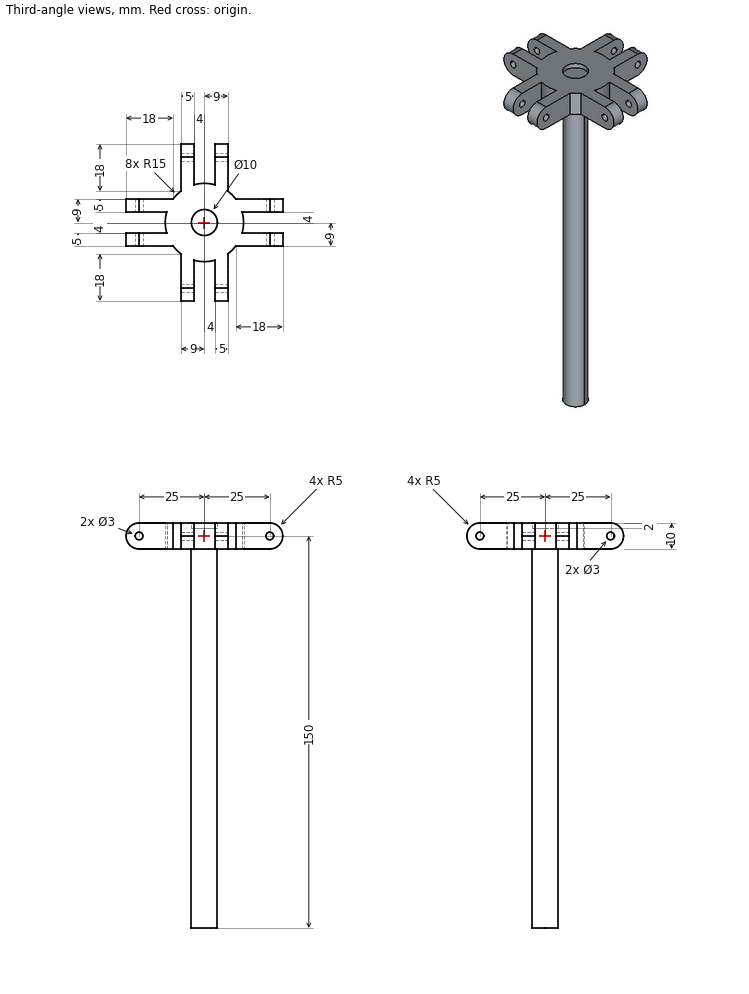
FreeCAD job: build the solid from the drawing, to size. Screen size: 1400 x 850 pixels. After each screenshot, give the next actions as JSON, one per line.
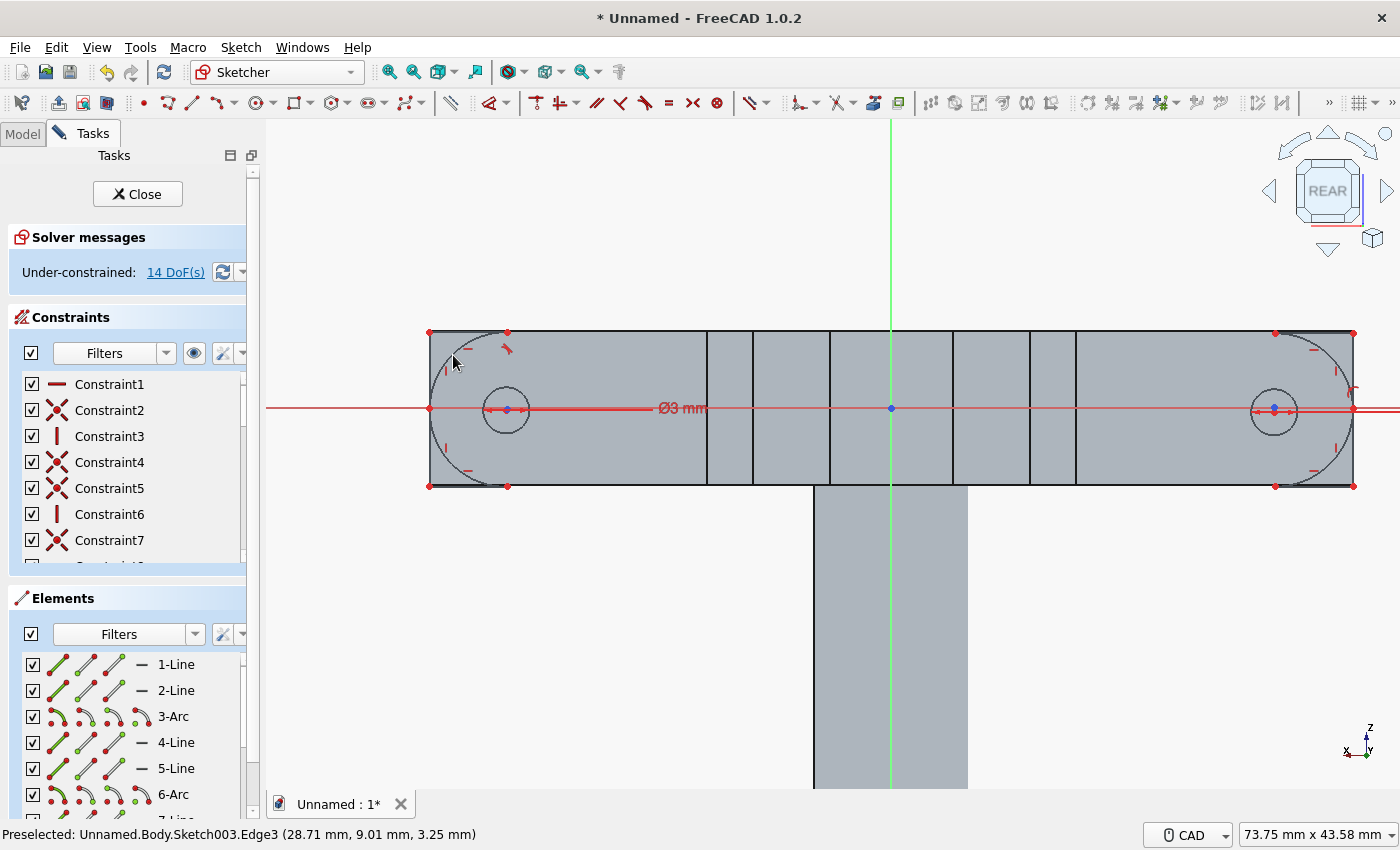
{"action": "left_click", "coordinate": [430, 355]}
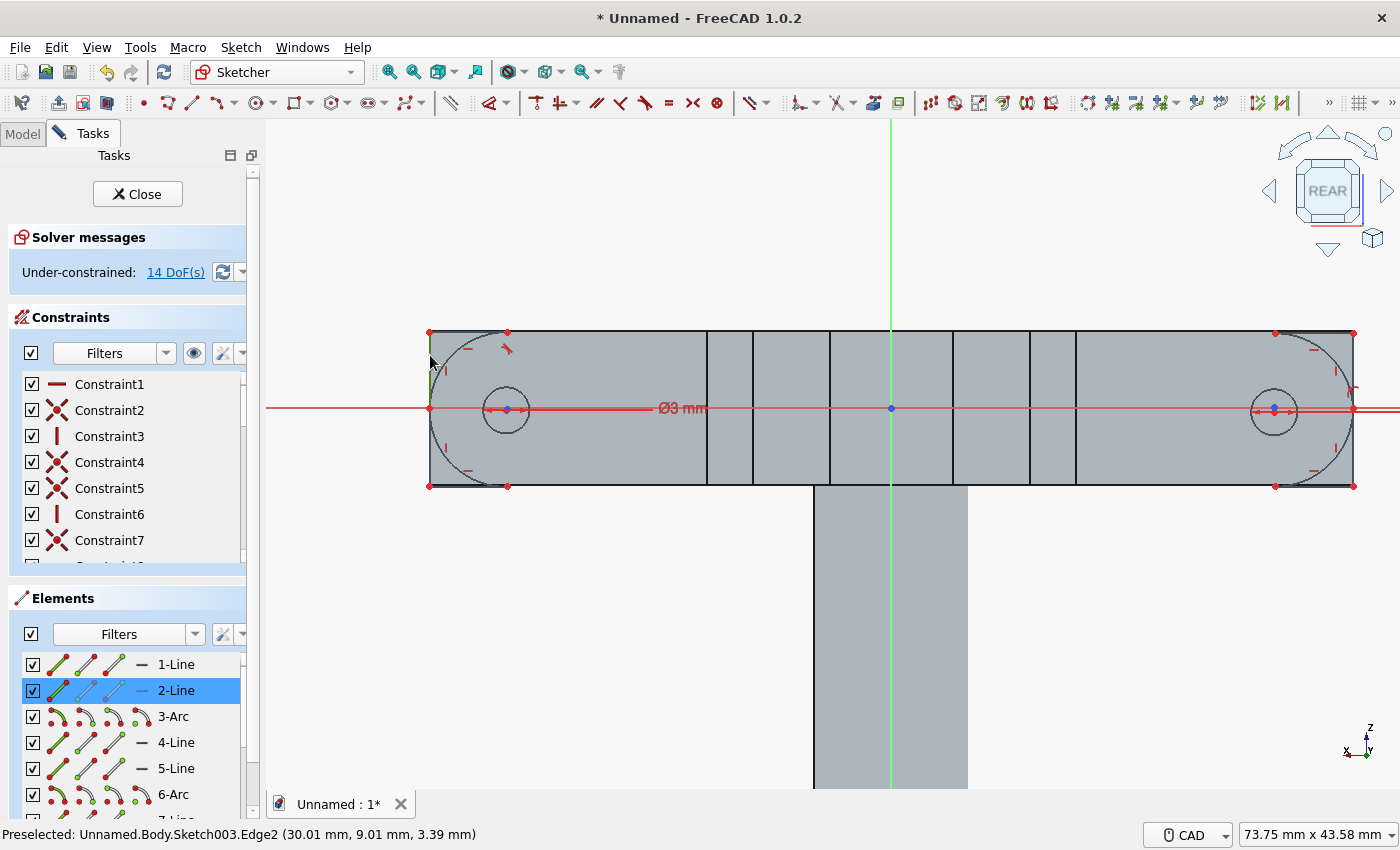
{"action": "left_click", "coordinate": [453, 354]}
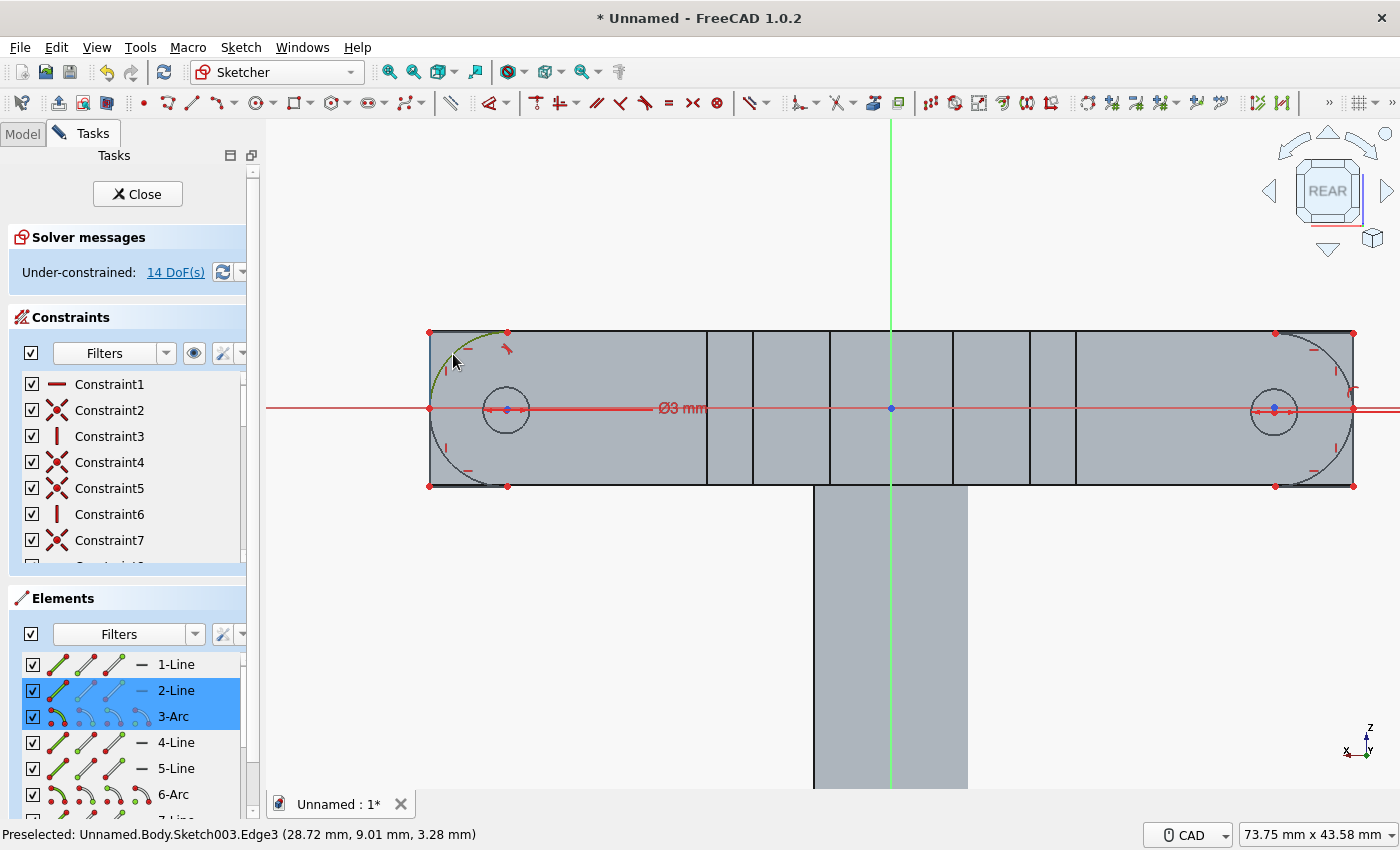
{"action": "key", "text": "t"}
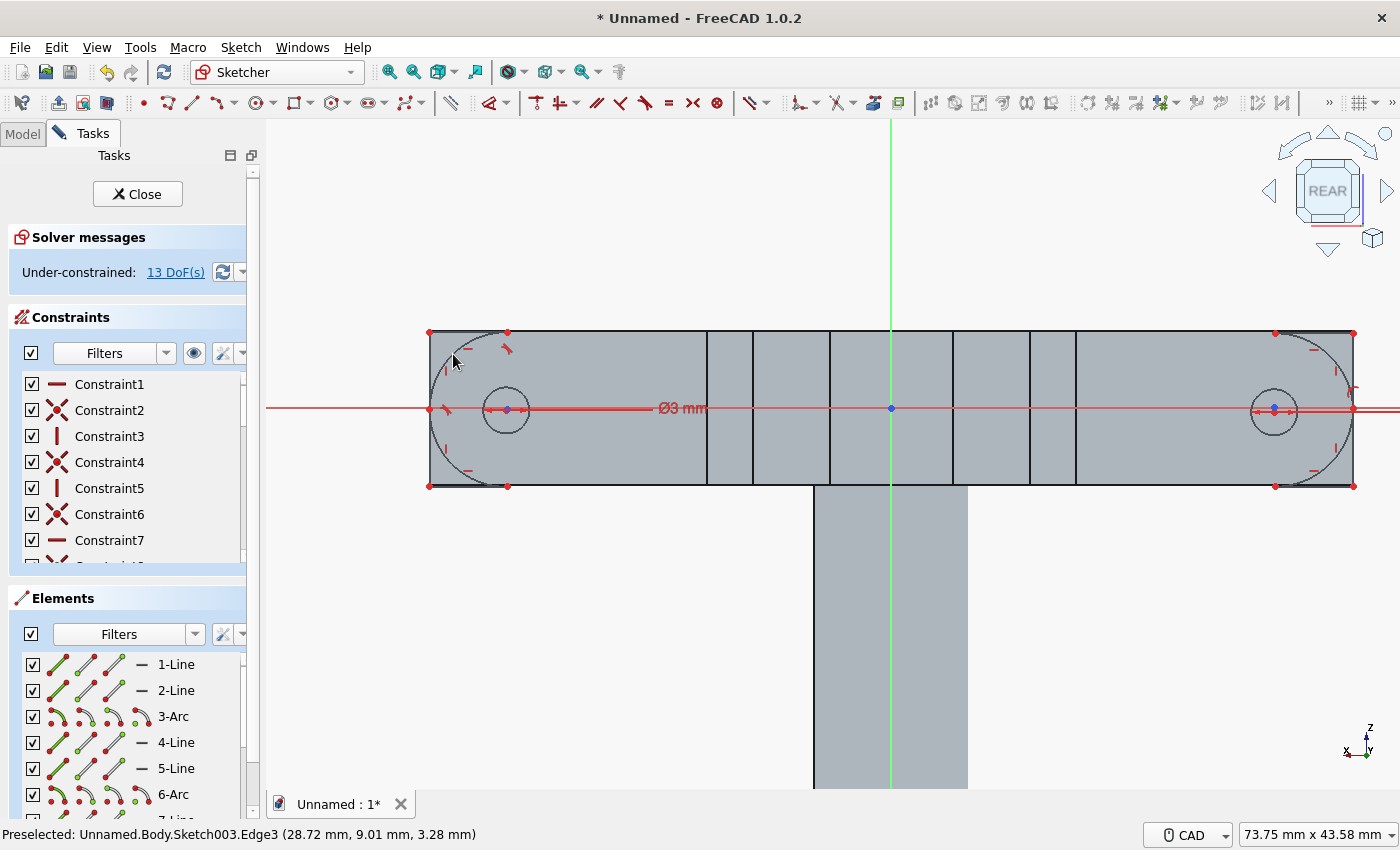
{"action": "left_click", "coordinate": [430, 355]}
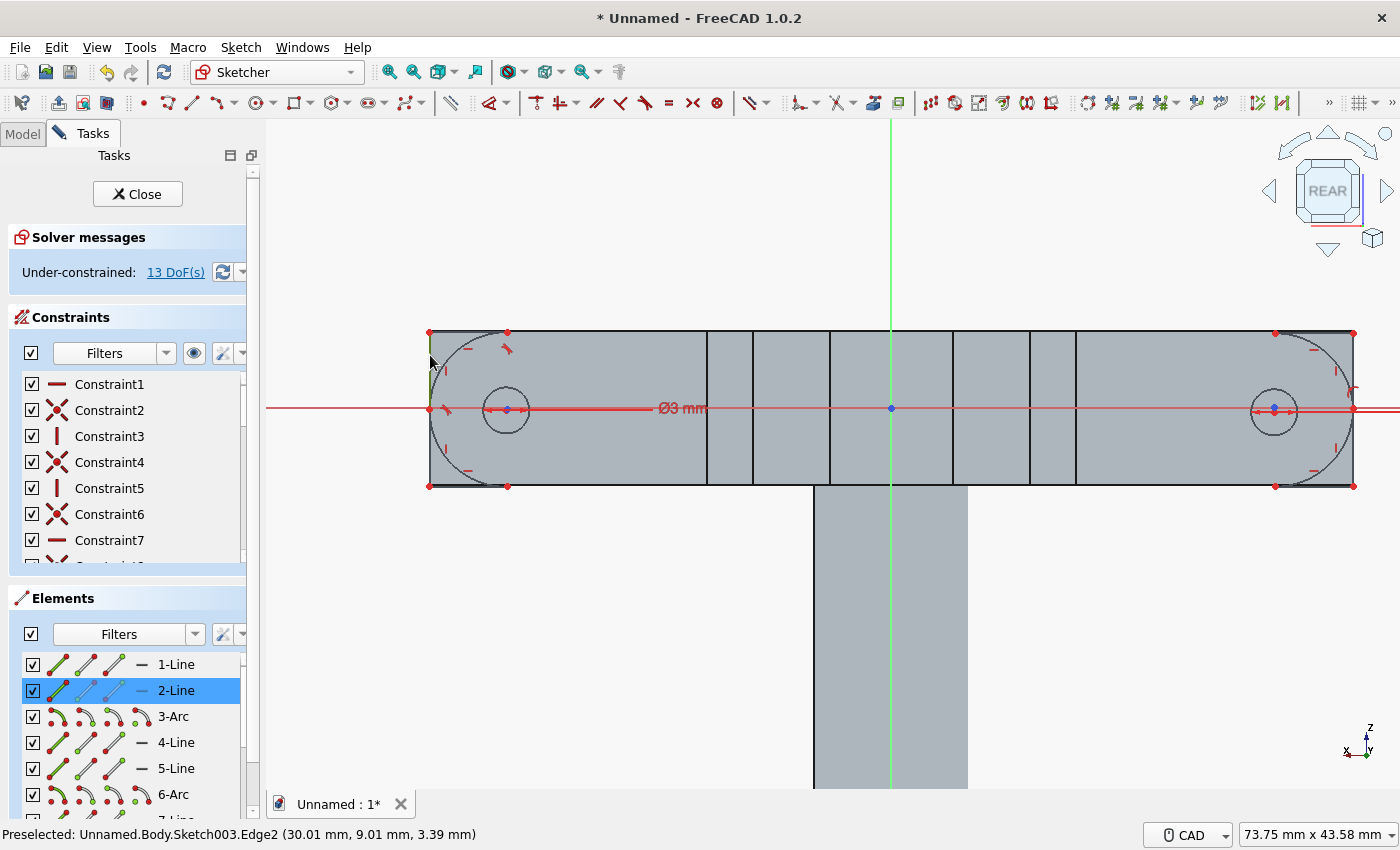
{"action": "left_click", "coordinate": [452, 465]}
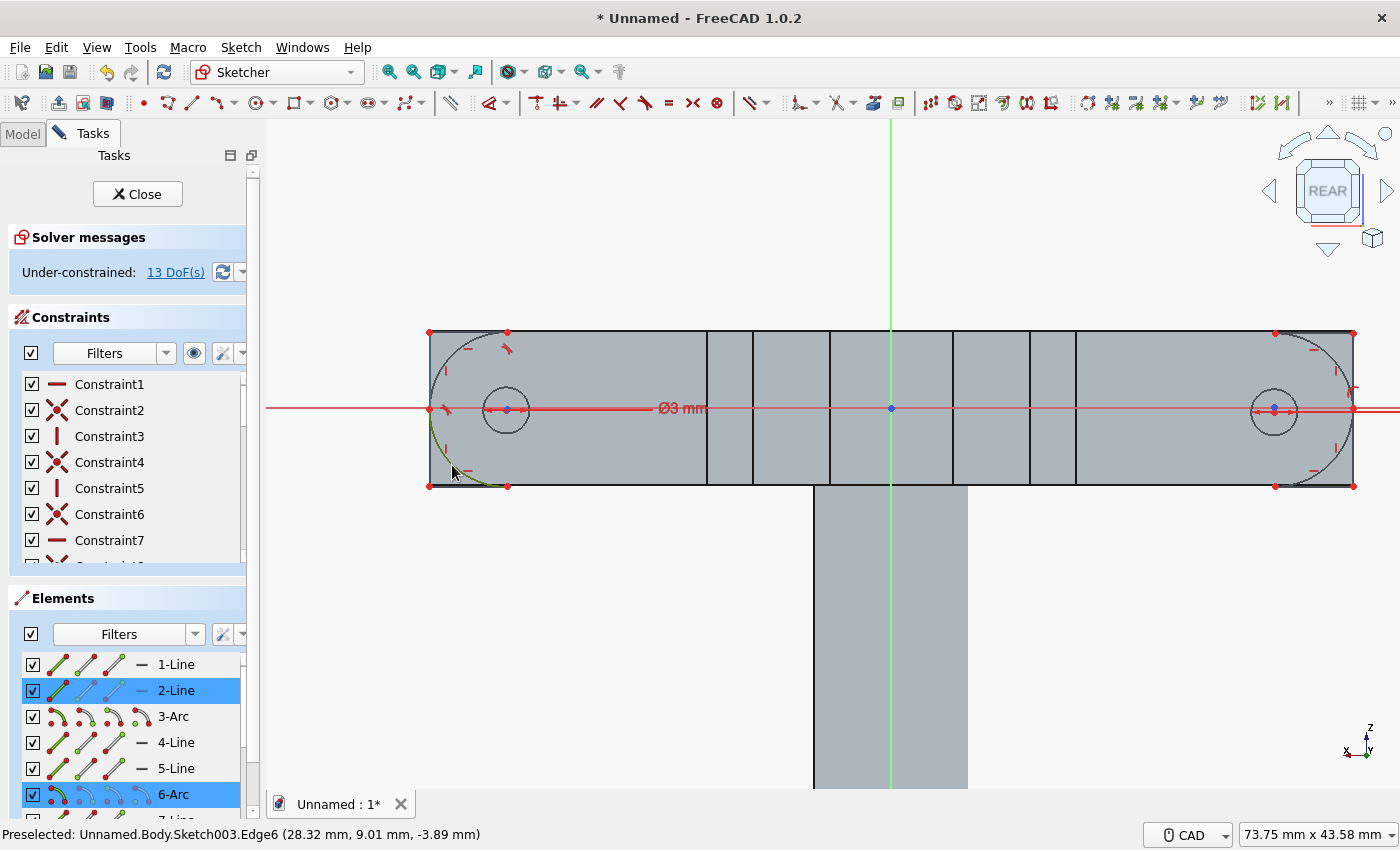
{"action": "key", "text": "t"}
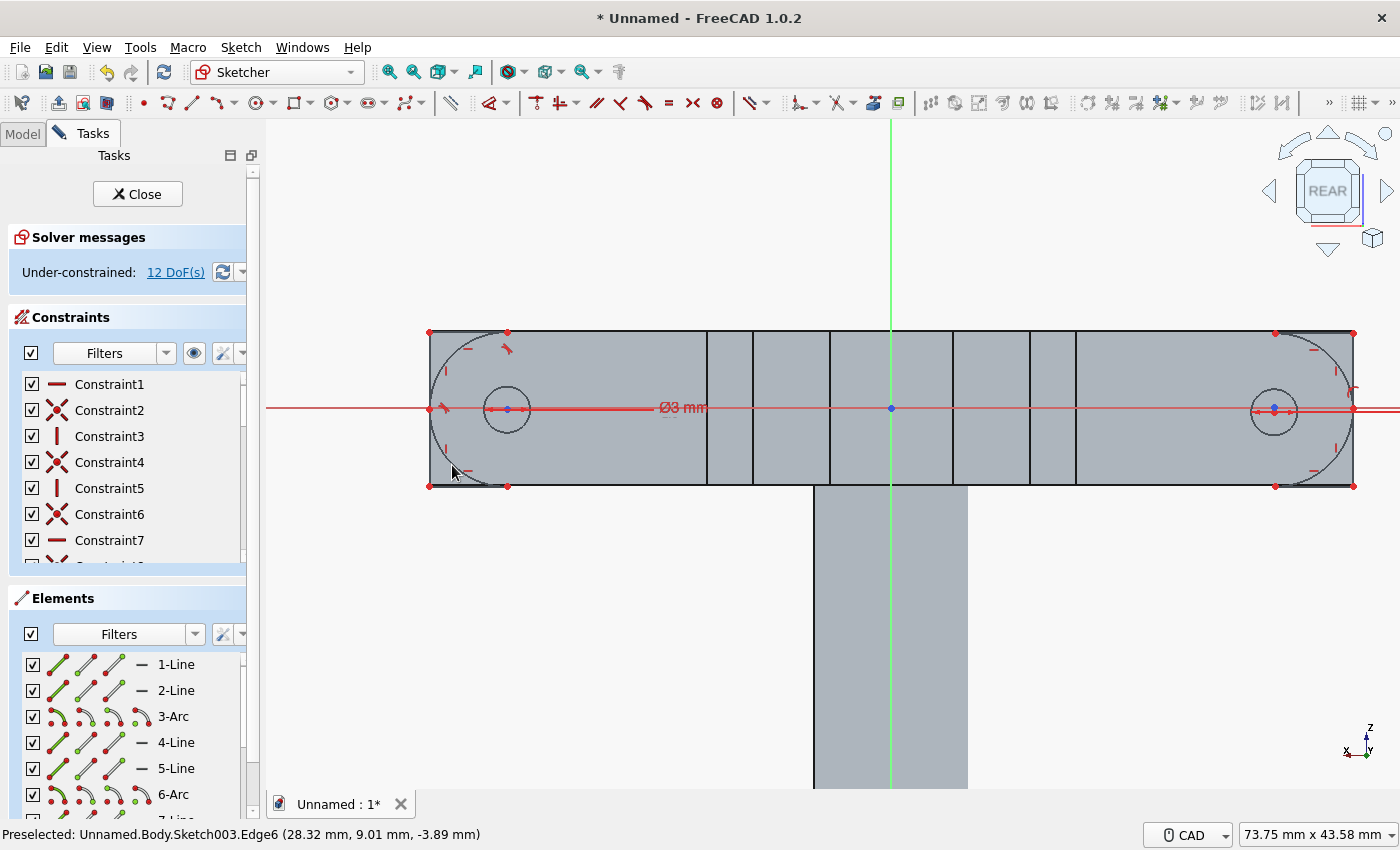
{"action": "left_click", "coordinate": [453, 487]}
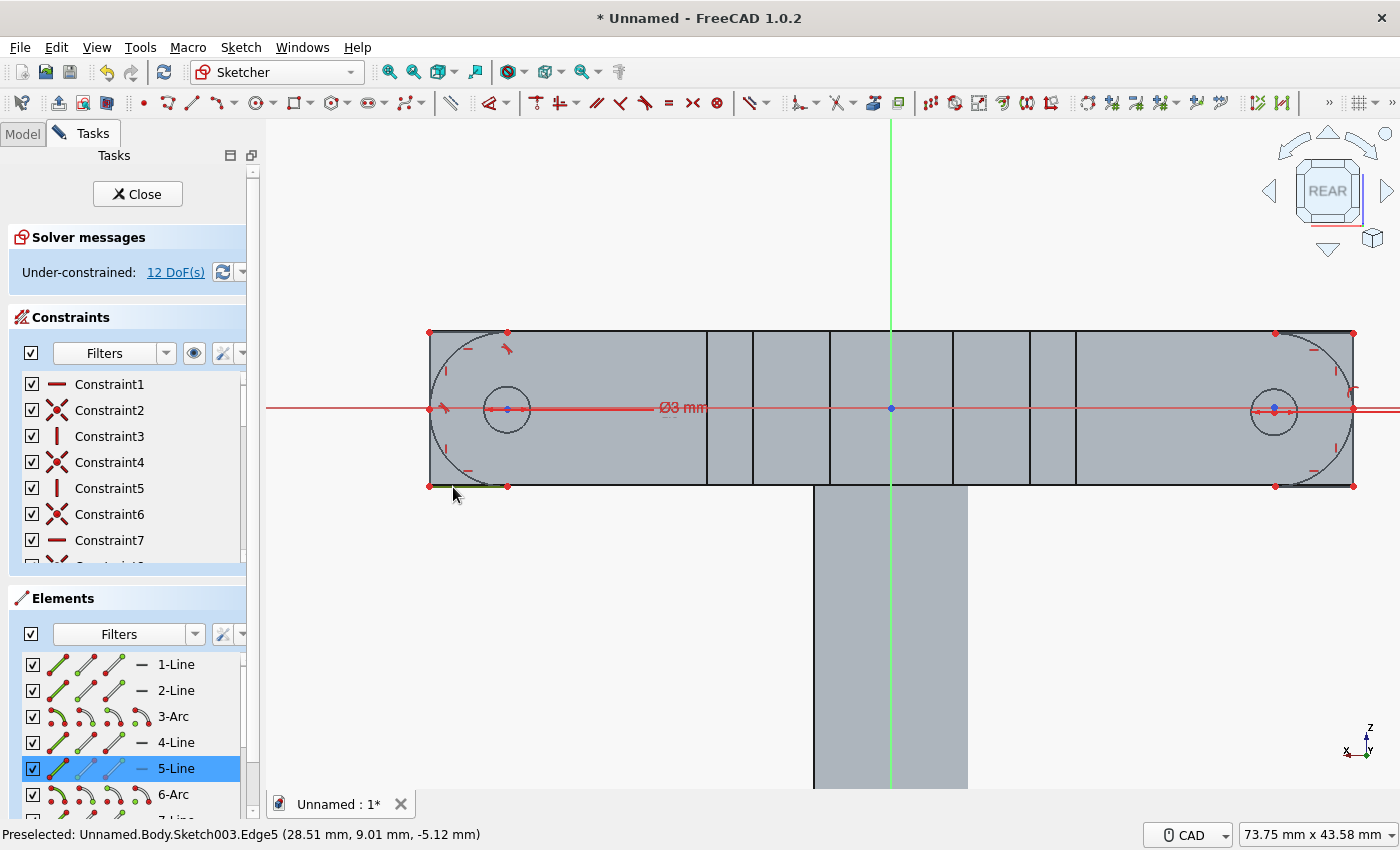
{"action": "left_click", "coordinate": [453, 464]}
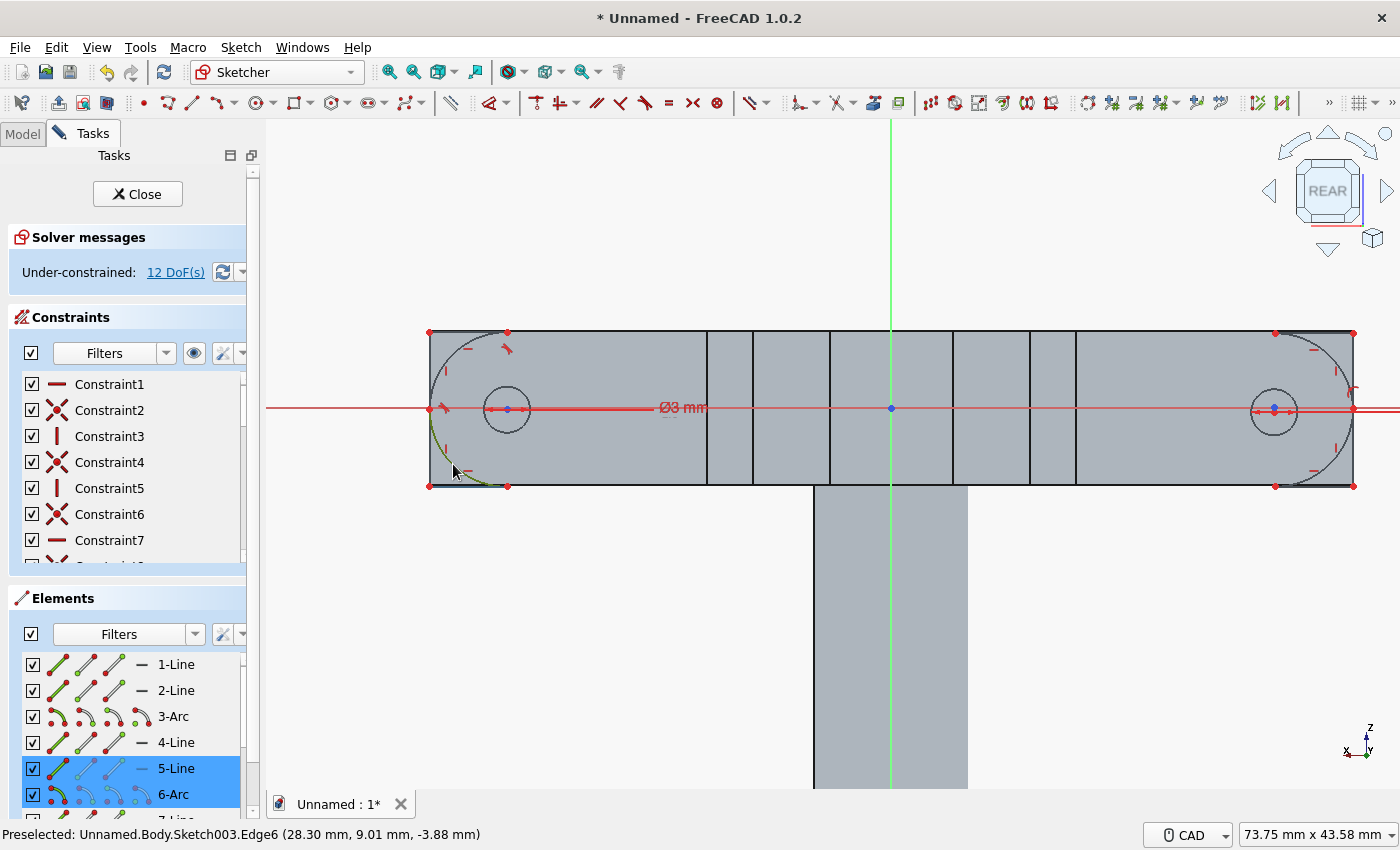
{"action": "left_click", "coordinate": [646, 104]}